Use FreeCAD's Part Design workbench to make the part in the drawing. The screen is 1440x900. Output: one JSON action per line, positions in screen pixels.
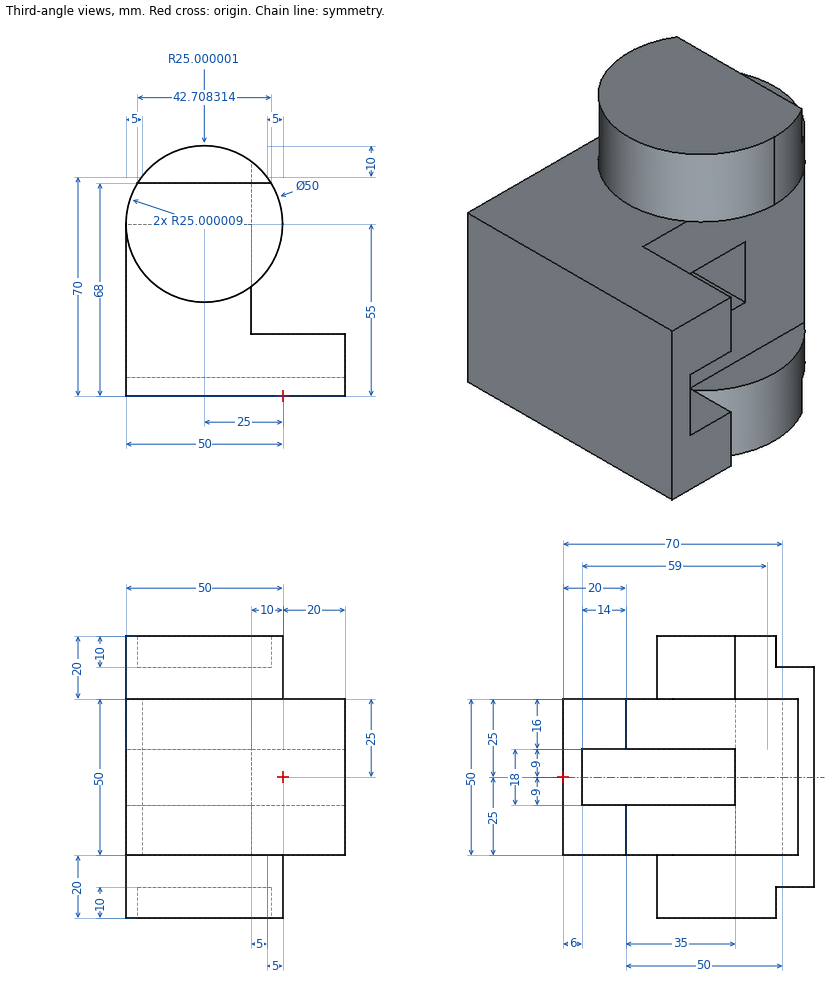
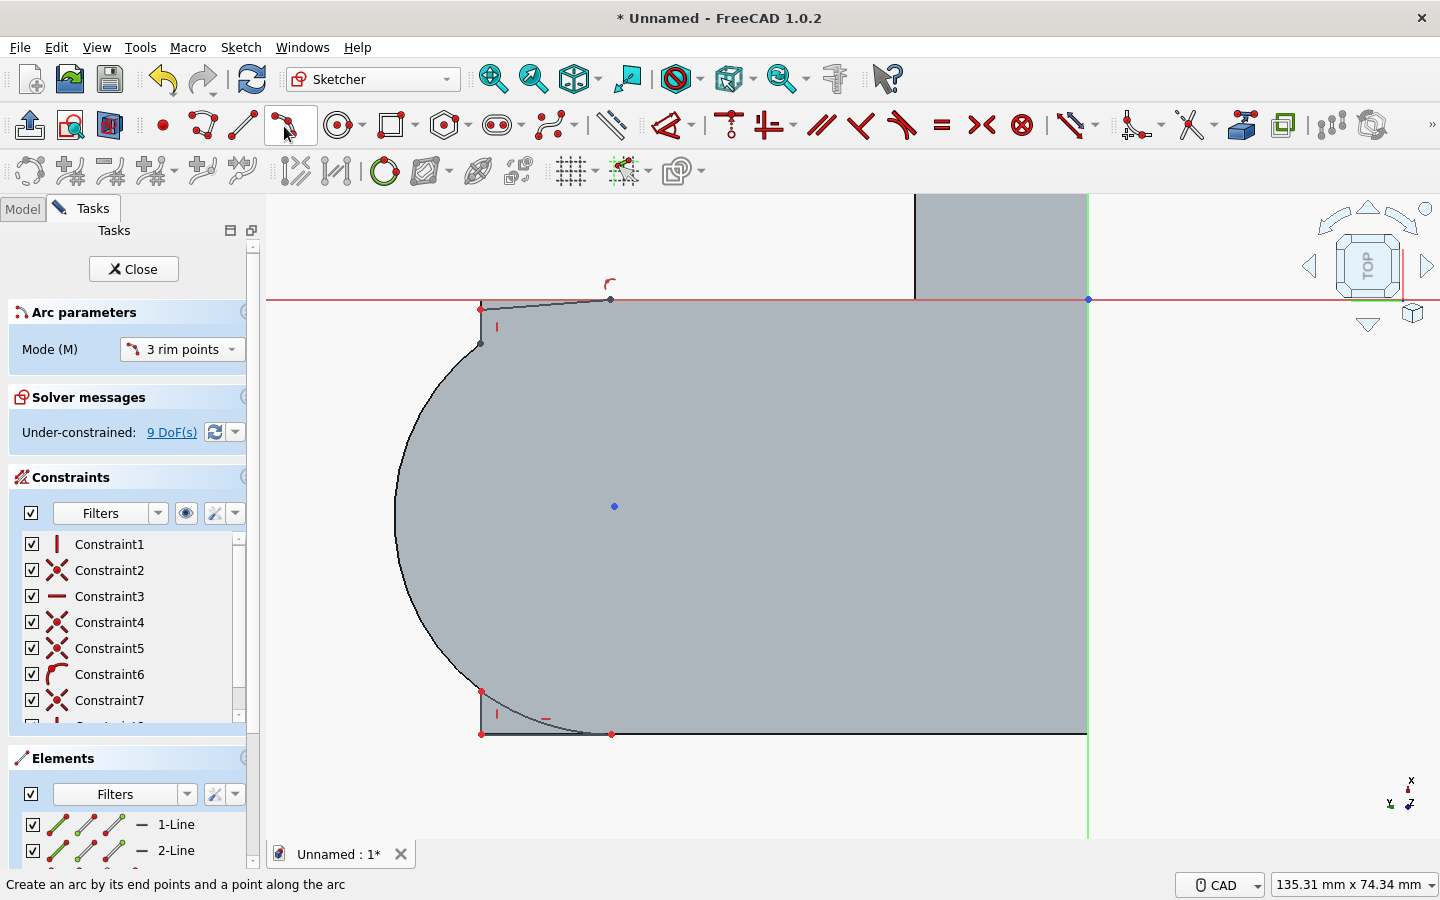
{"action": "left_click", "coordinate": [481, 344]}
{"action": "left_click", "coordinate": [611, 300]}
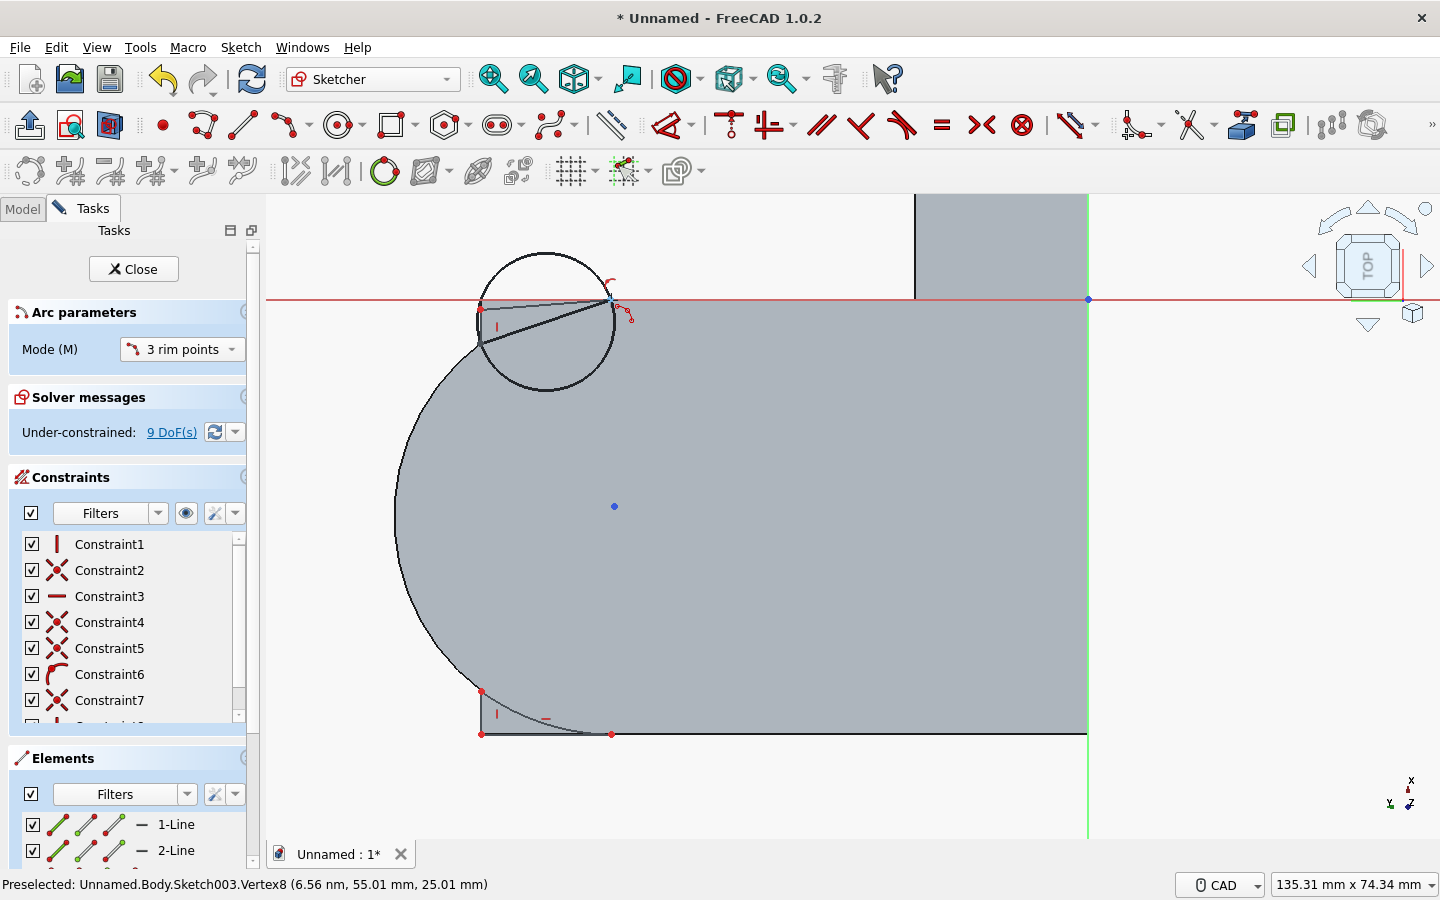
{"action": "scroll", "coordinate": [542, 311], "scroll_direction": "up", "scroll_amount": 2}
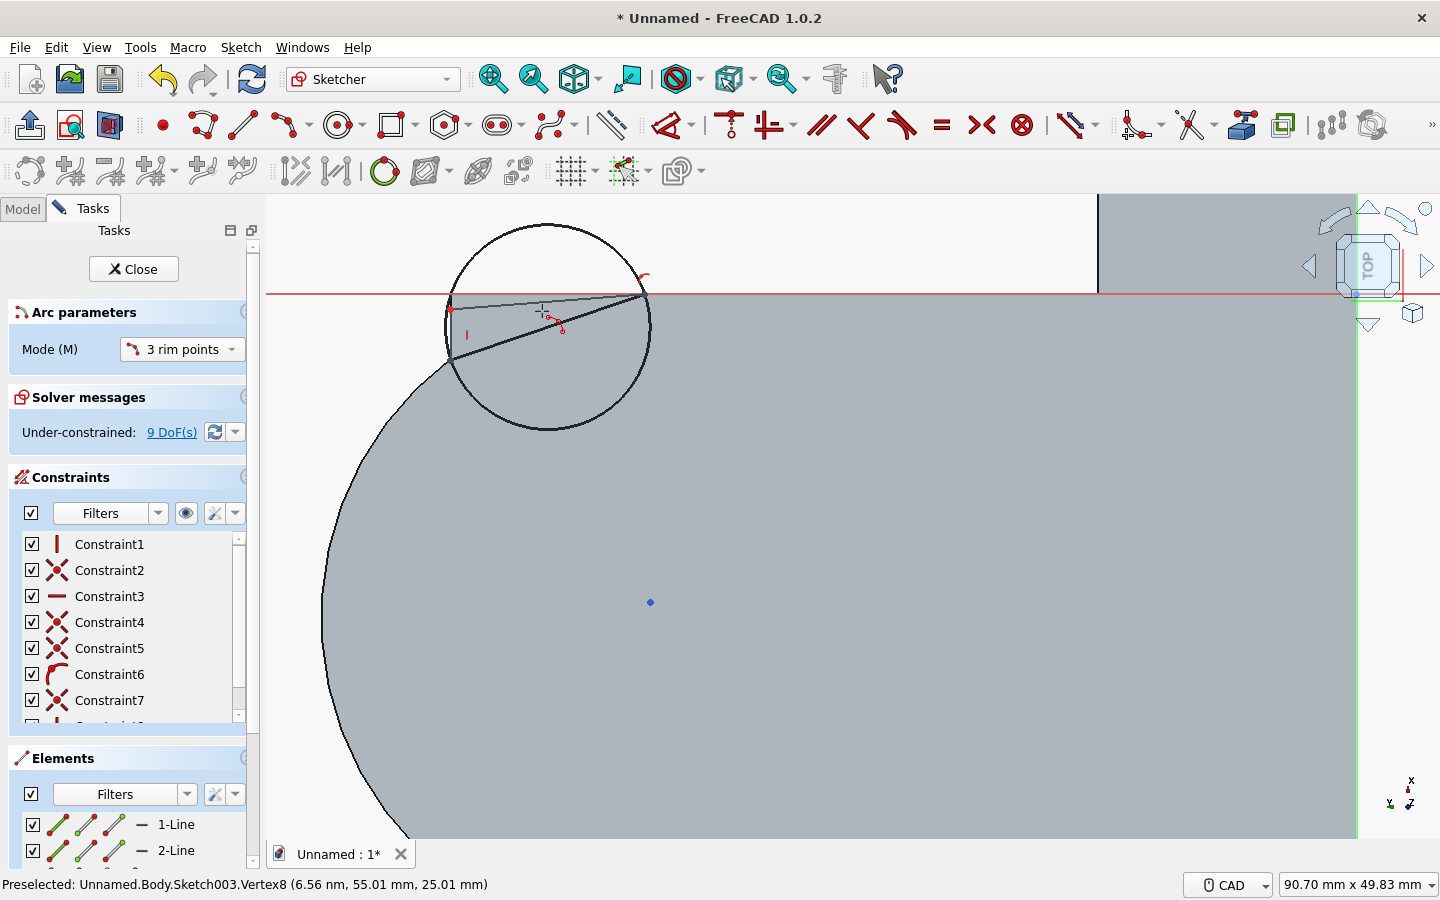
{"action": "left_click", "coordinate": [543, 311]}
{"action": "key", "text": "Escape"}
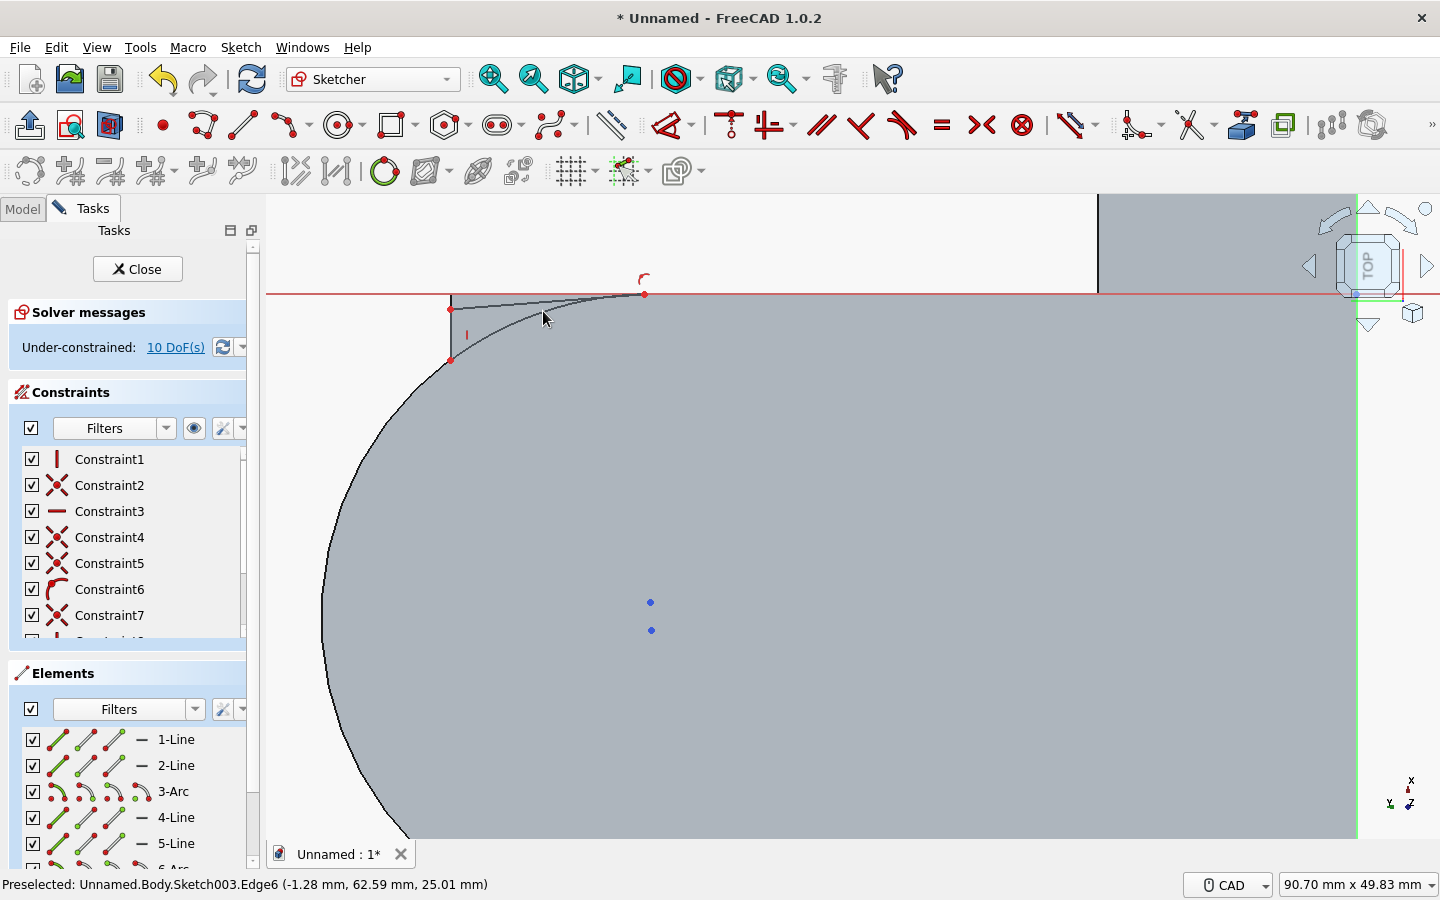
{"action": "scroll", "coordinate": [542, 310], "scroll_direction": "down", "scroll_amount": 2}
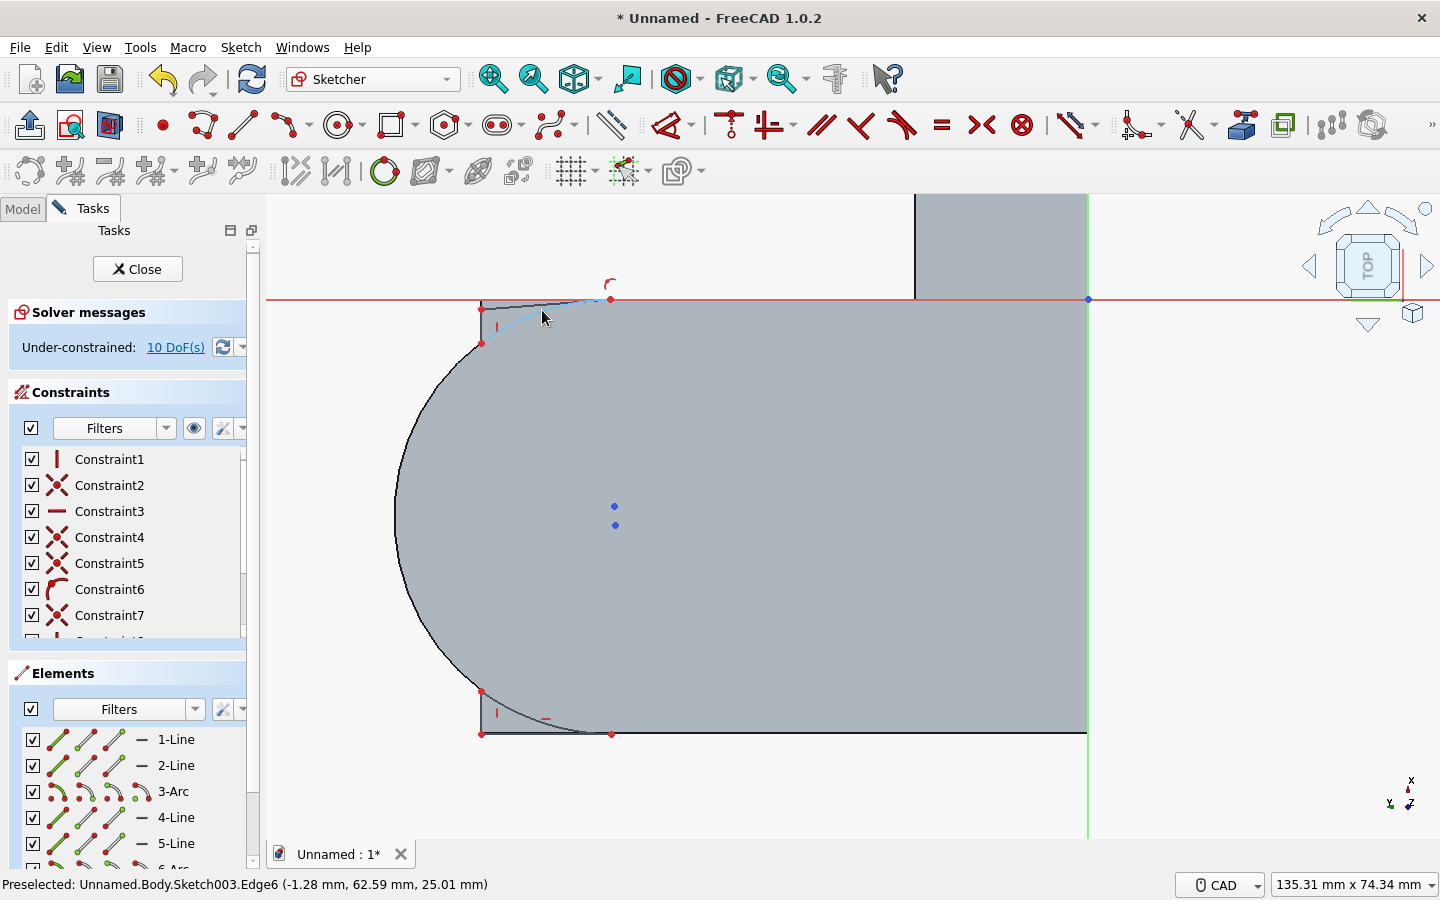
{"action": "left_click", "coordinate": [520, 734]}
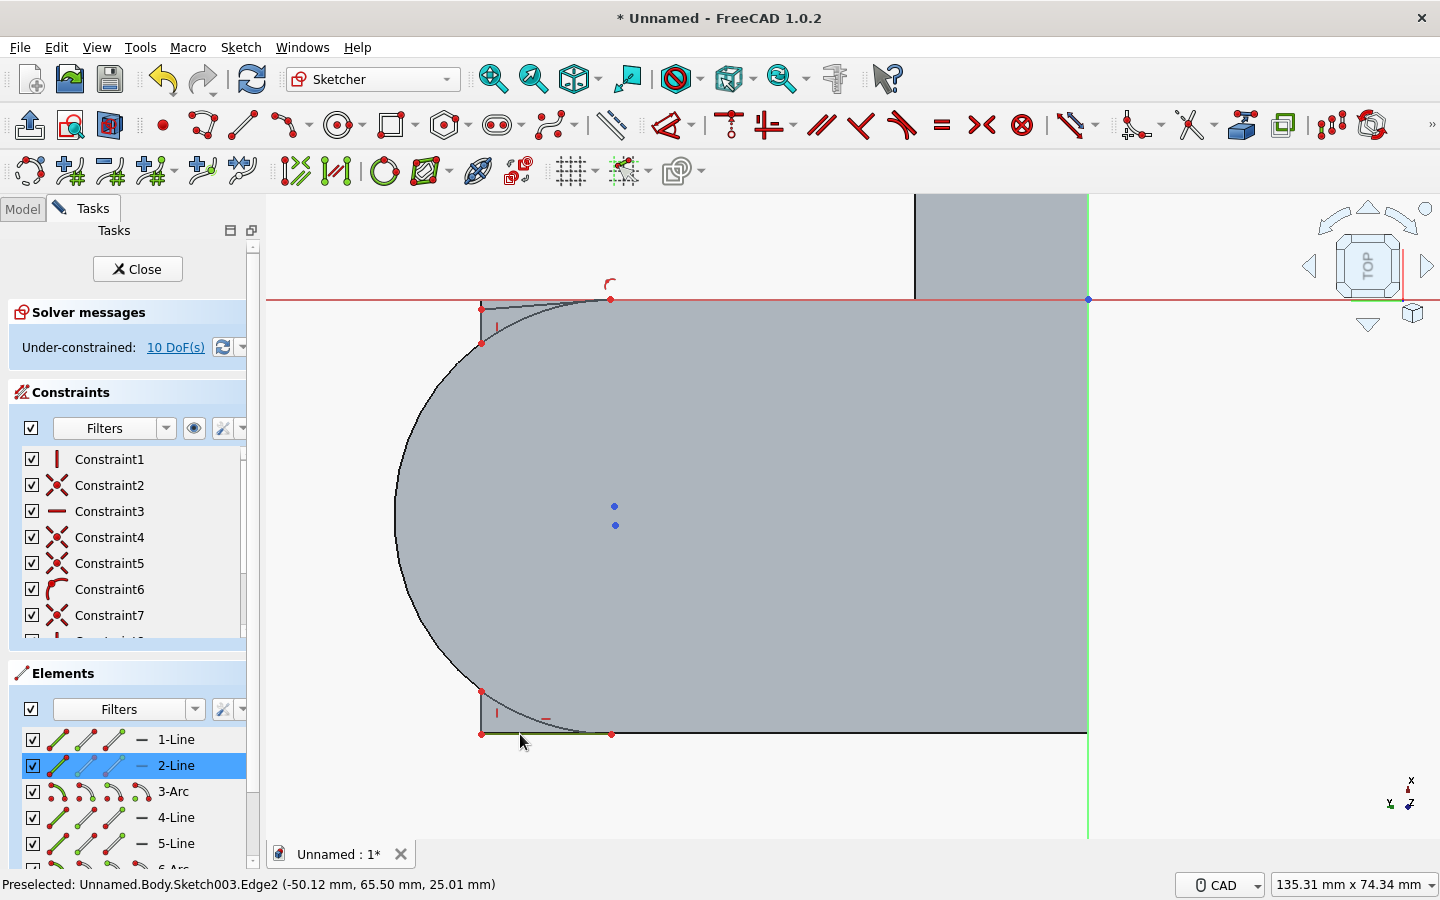
{"action": "left_click", "coordinate": [517, 712]}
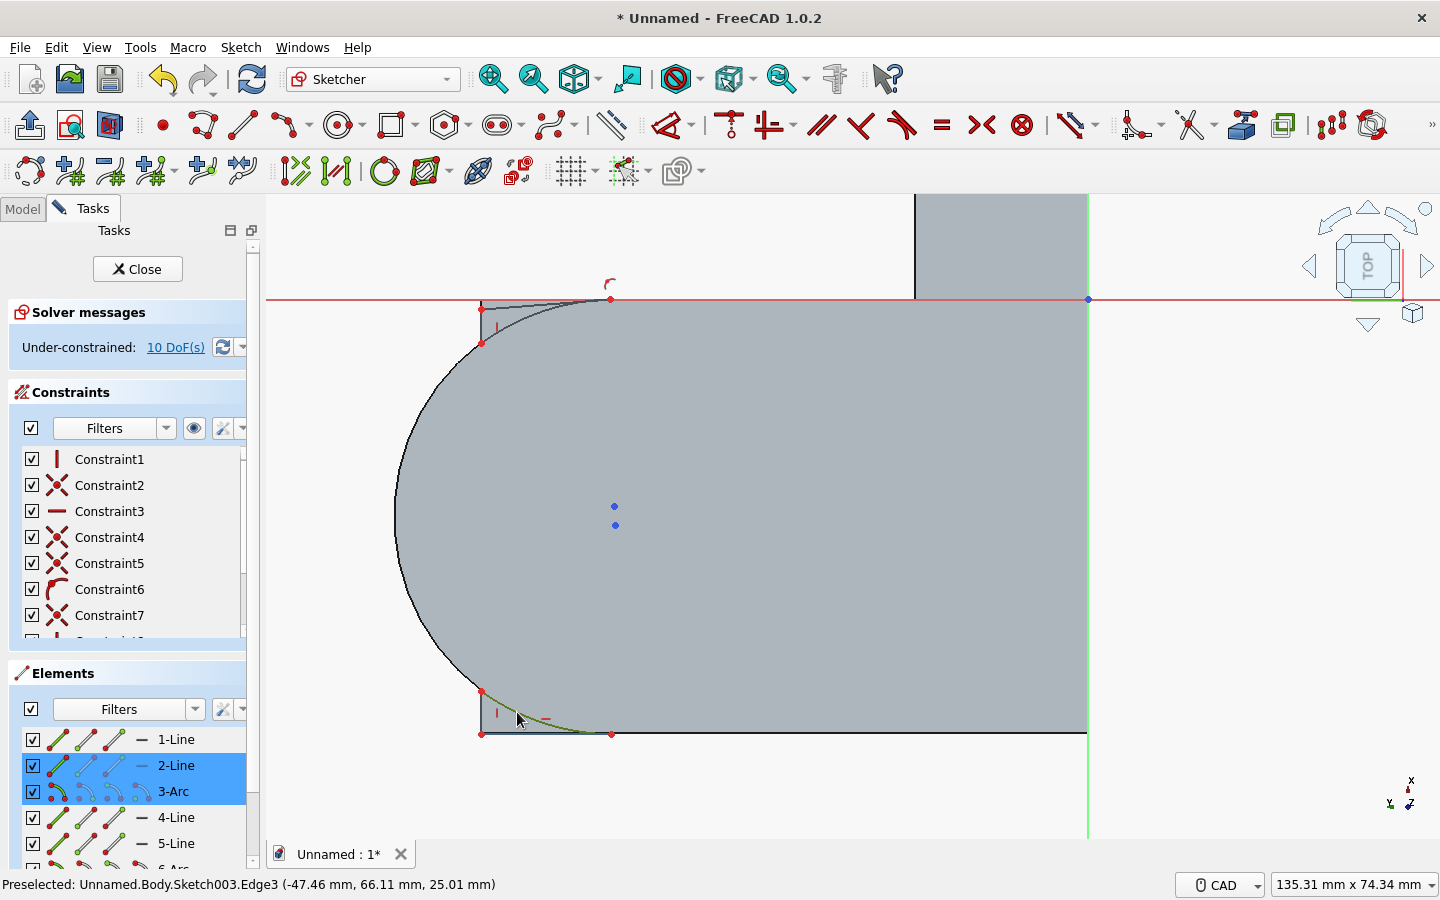
{"action": "left_click", "coordinate": [902, 126]}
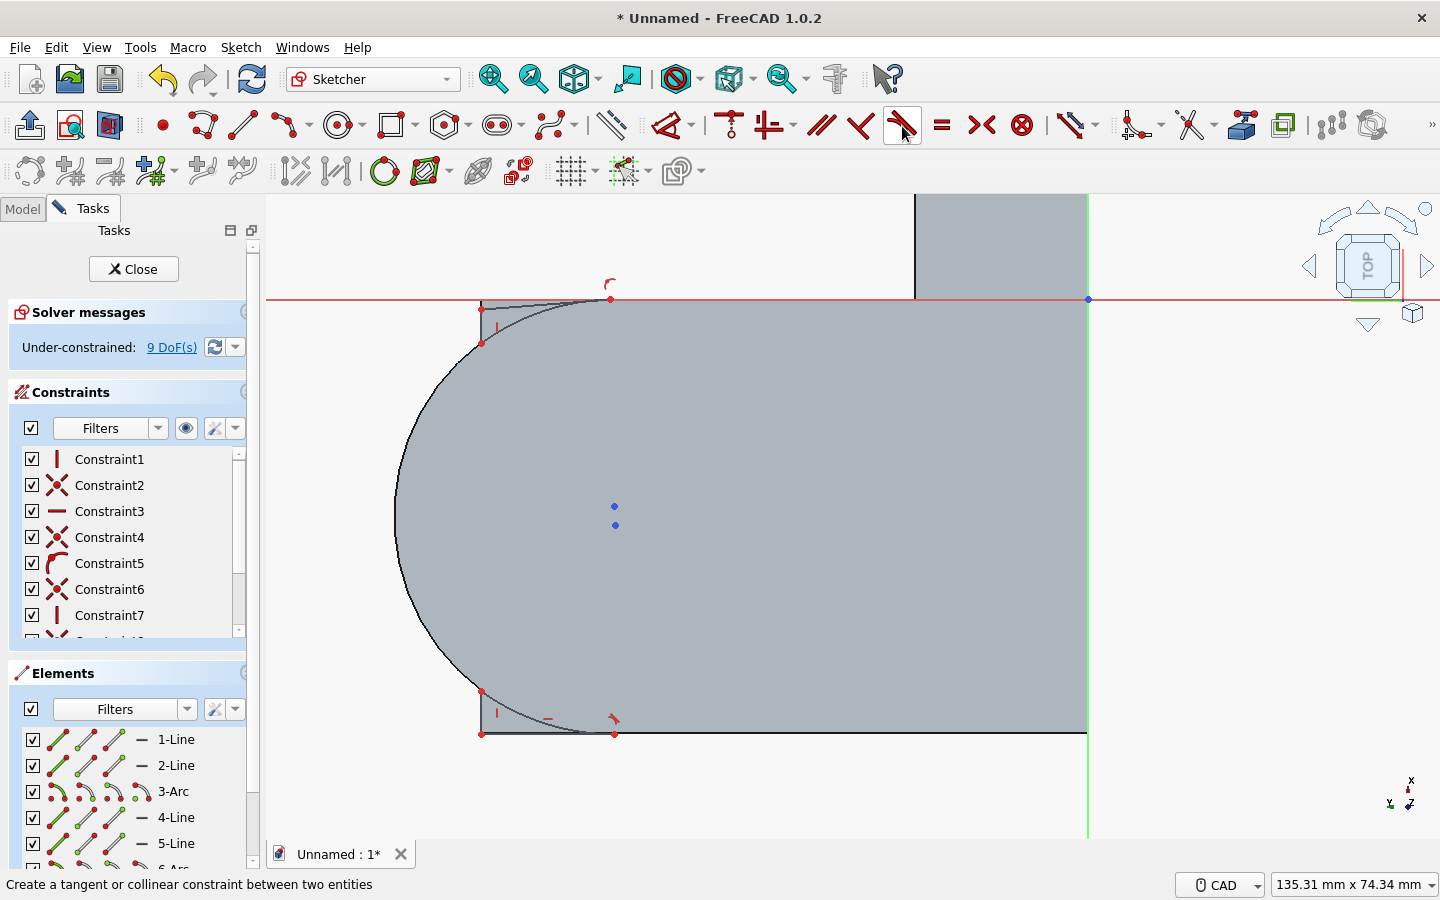
{"action": "scroll", "coordinate": [507, 308], "scroll_direction": "up", "scroll_amount": 3}